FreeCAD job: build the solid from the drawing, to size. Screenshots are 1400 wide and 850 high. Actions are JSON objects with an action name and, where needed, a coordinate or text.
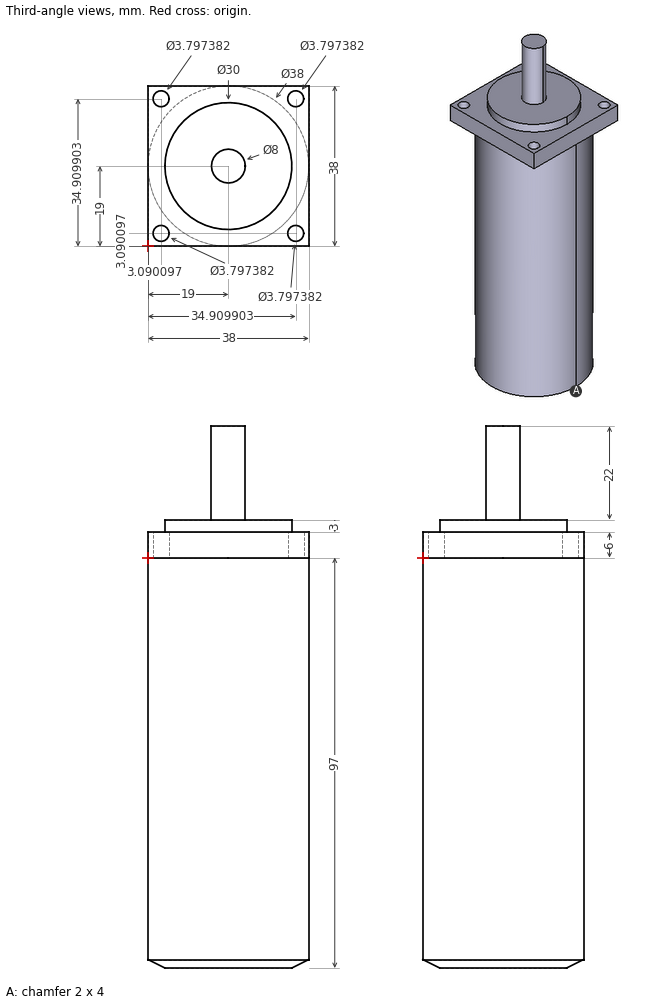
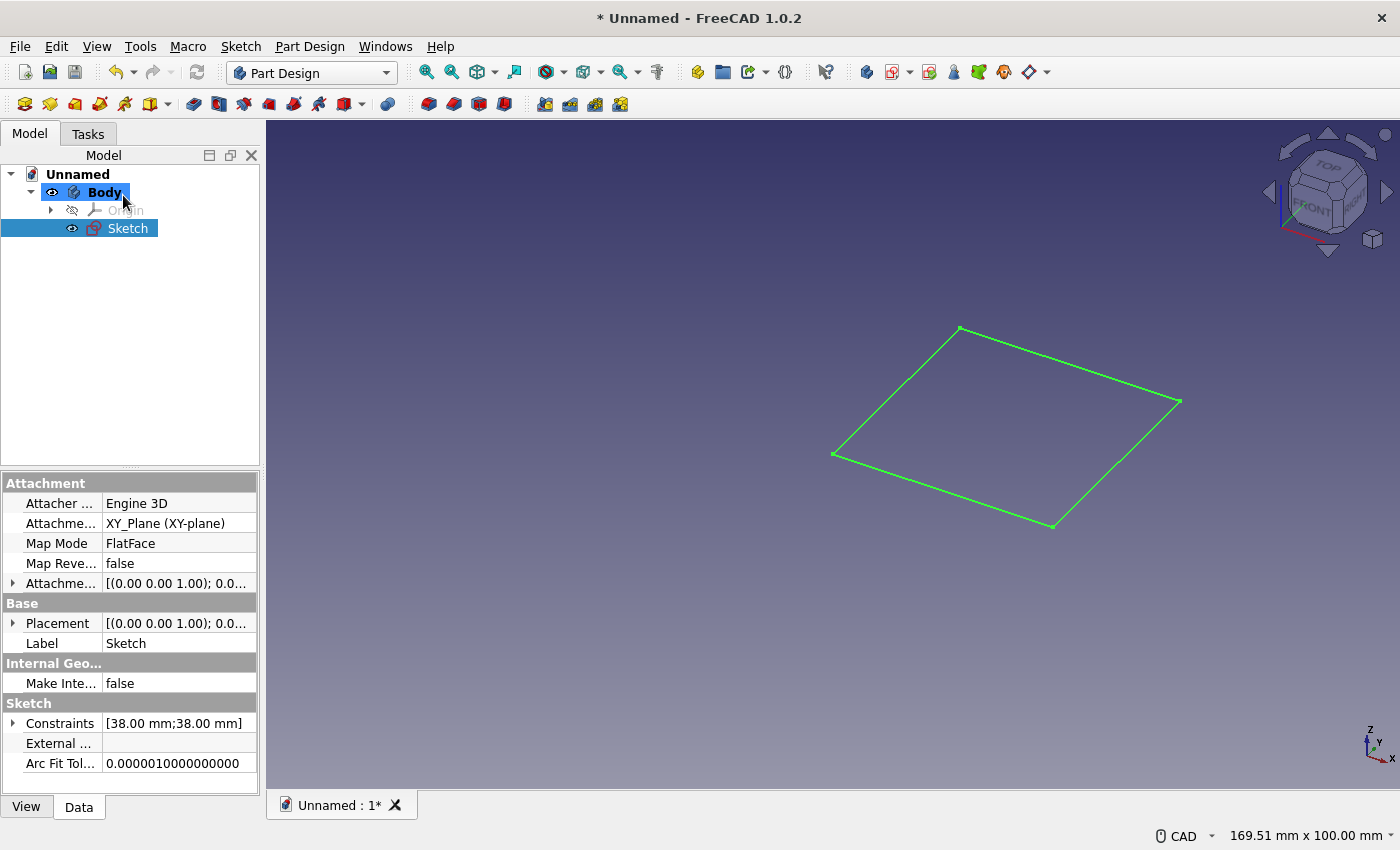
{"action": "left_click", "coordinate": [25, 104]}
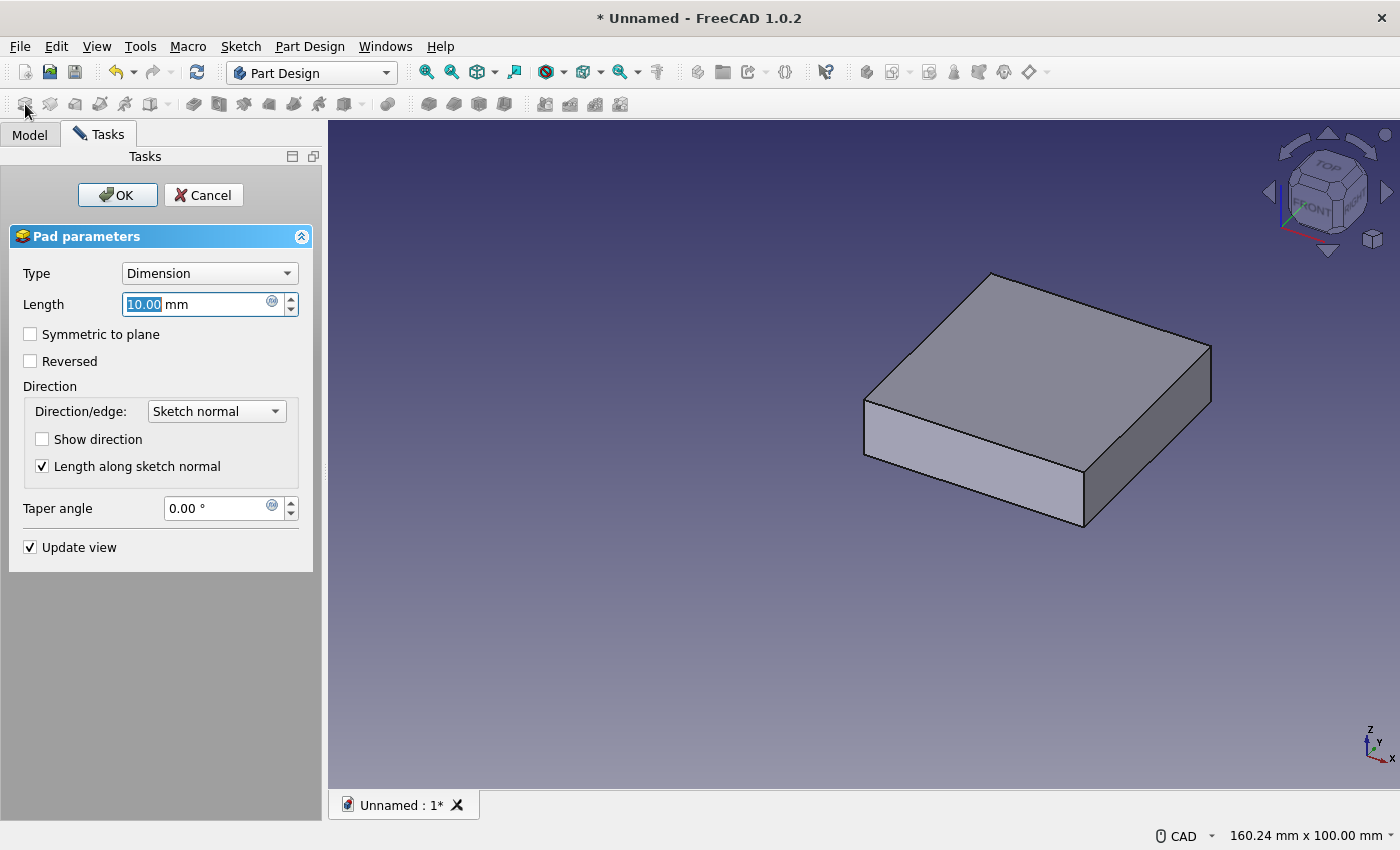
{"action": "type", "text": "6"}
{"action": "key", "text": "Tab"}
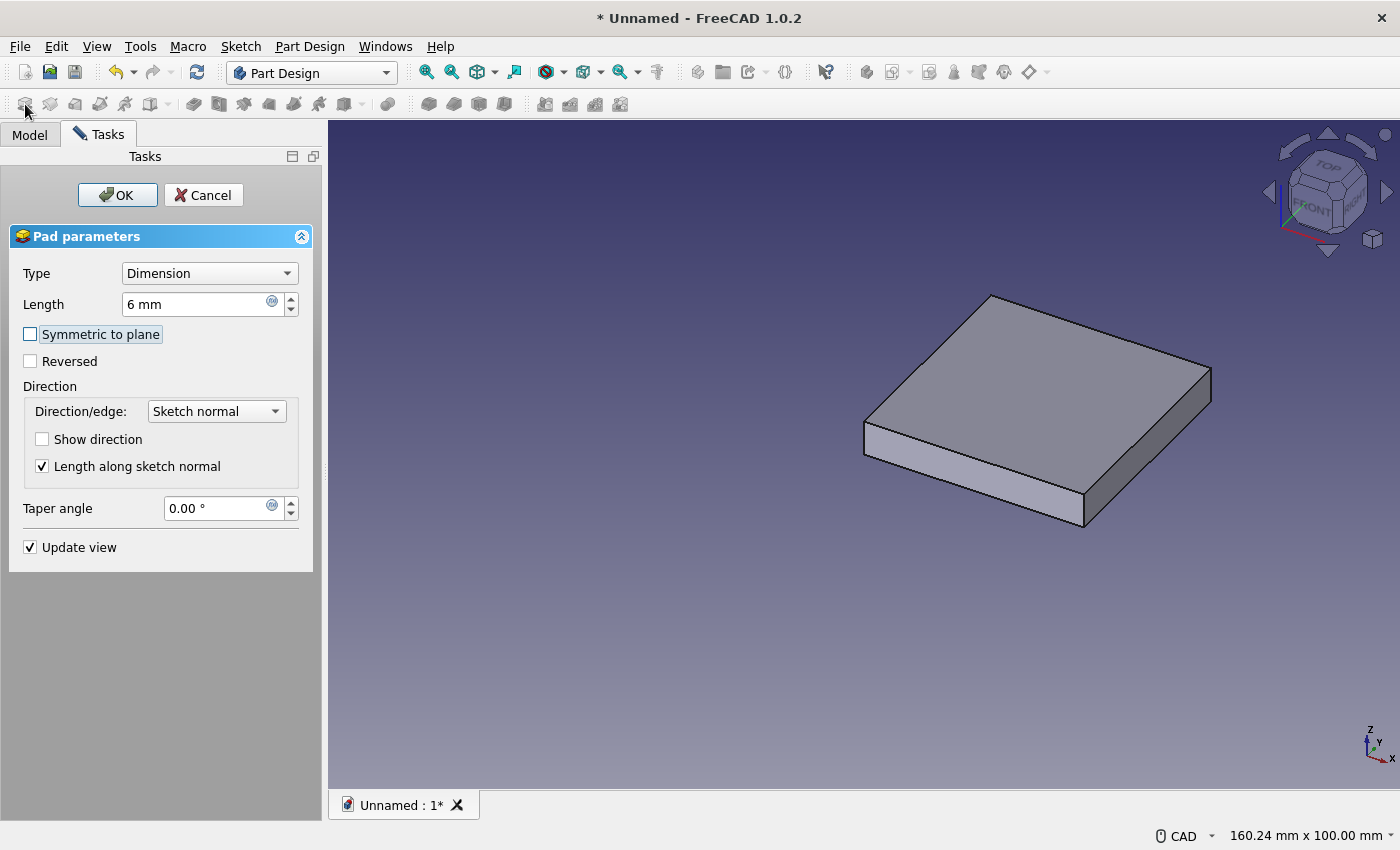
{"action": "left_click", "coordinate": [118, 195]}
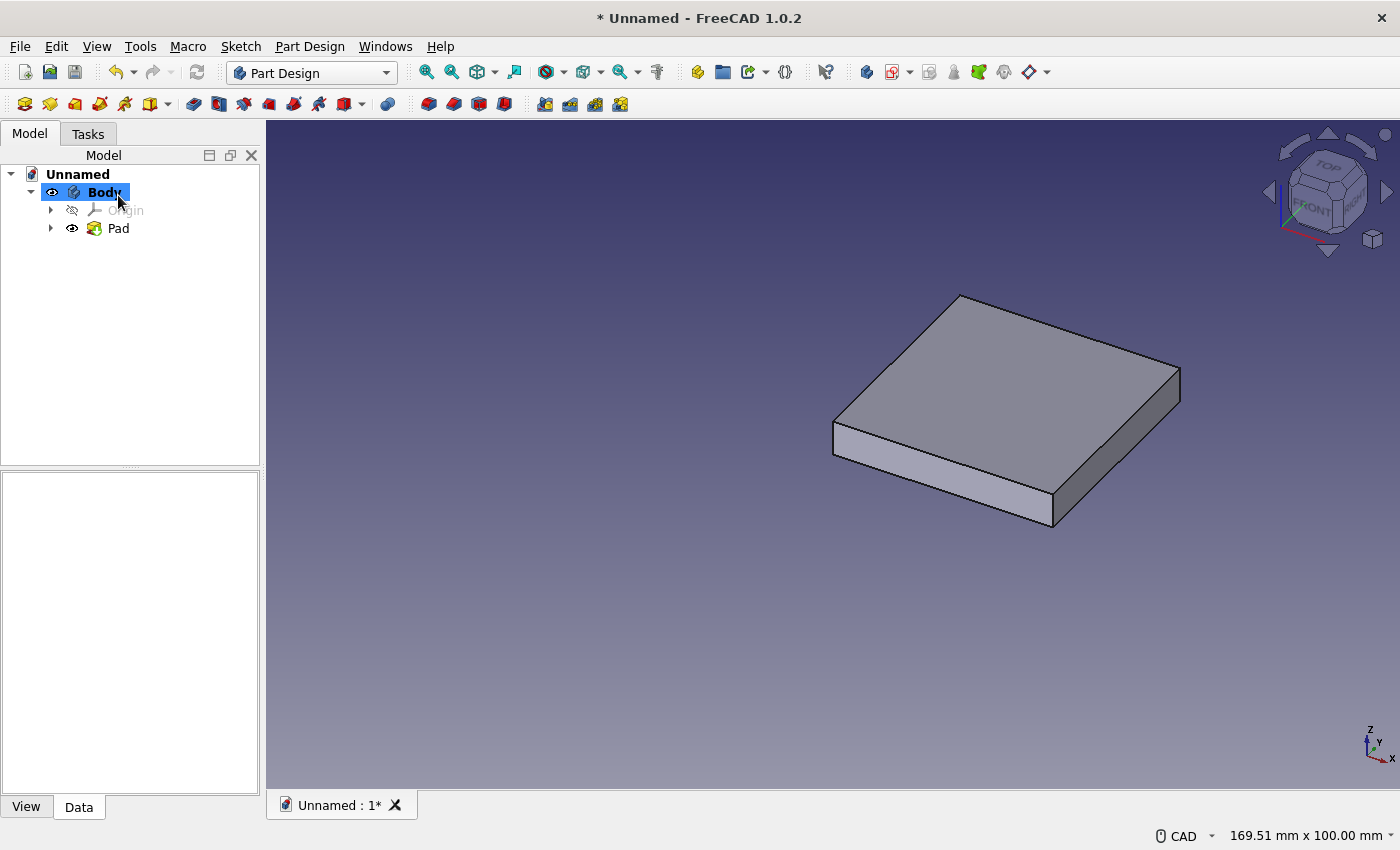
{"action": "key", "text": "v f"}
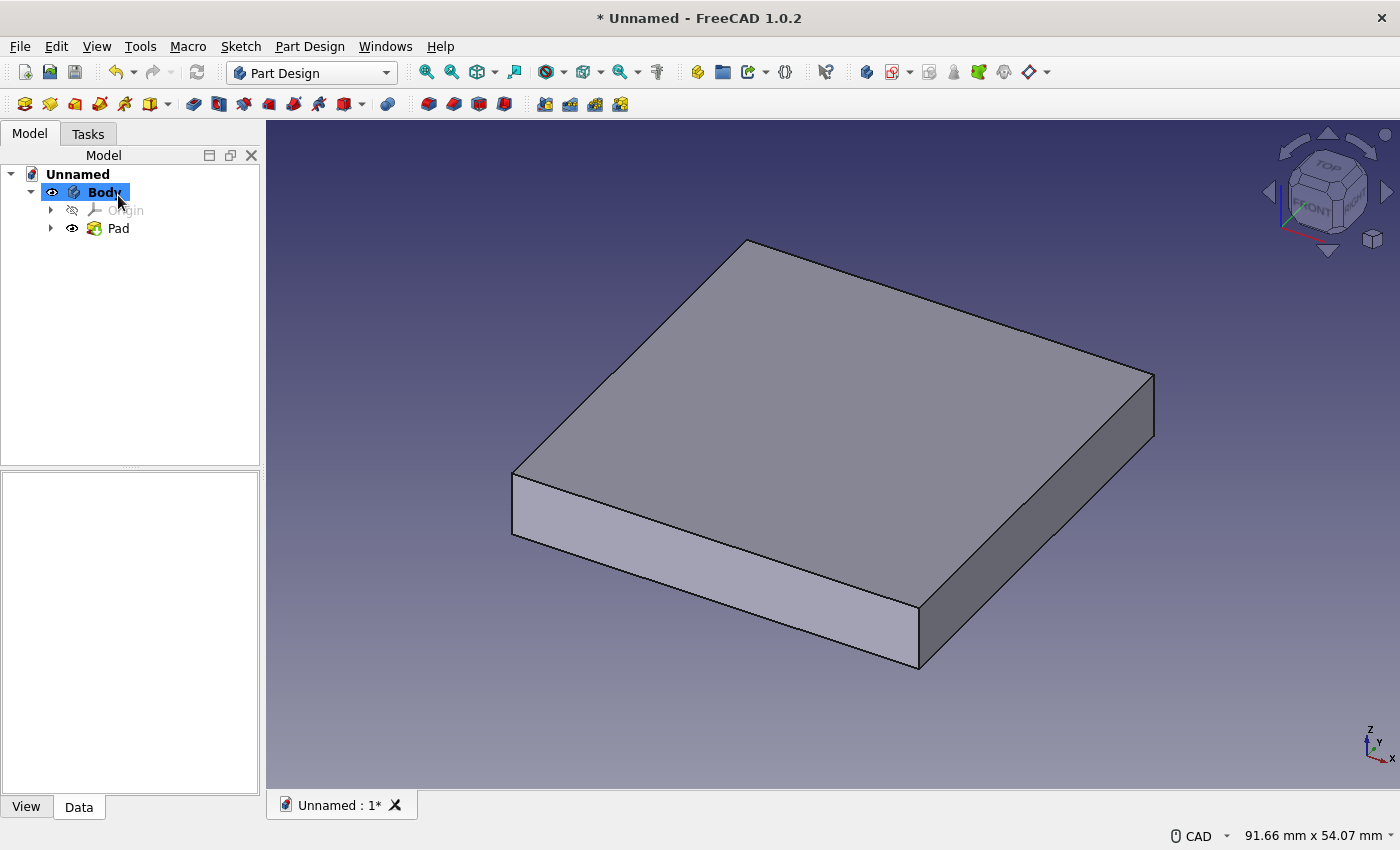
{"action": "left_click", "coordinate": [833, 423]}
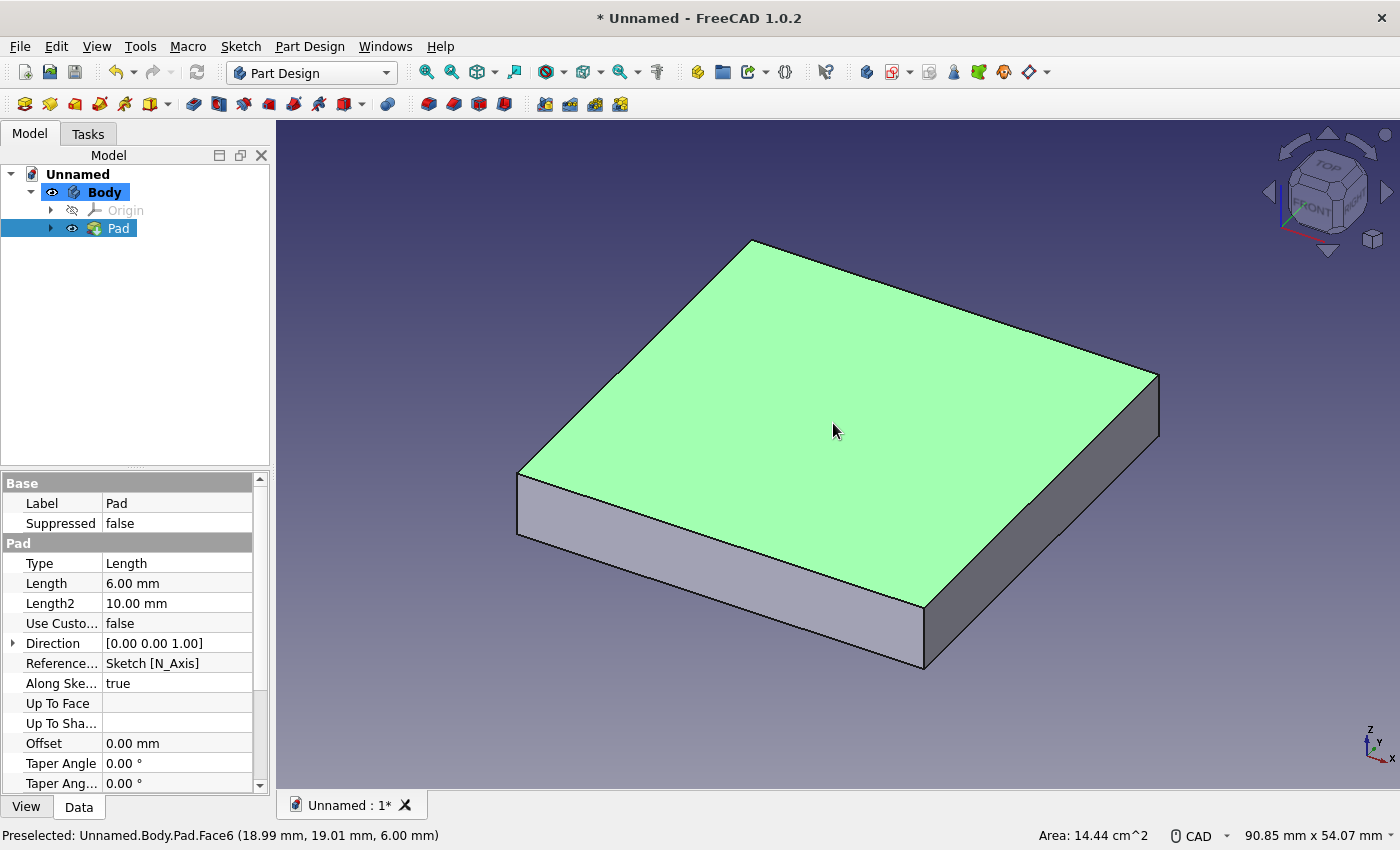
{"action": "left_click", "coordinate": [892, 72]}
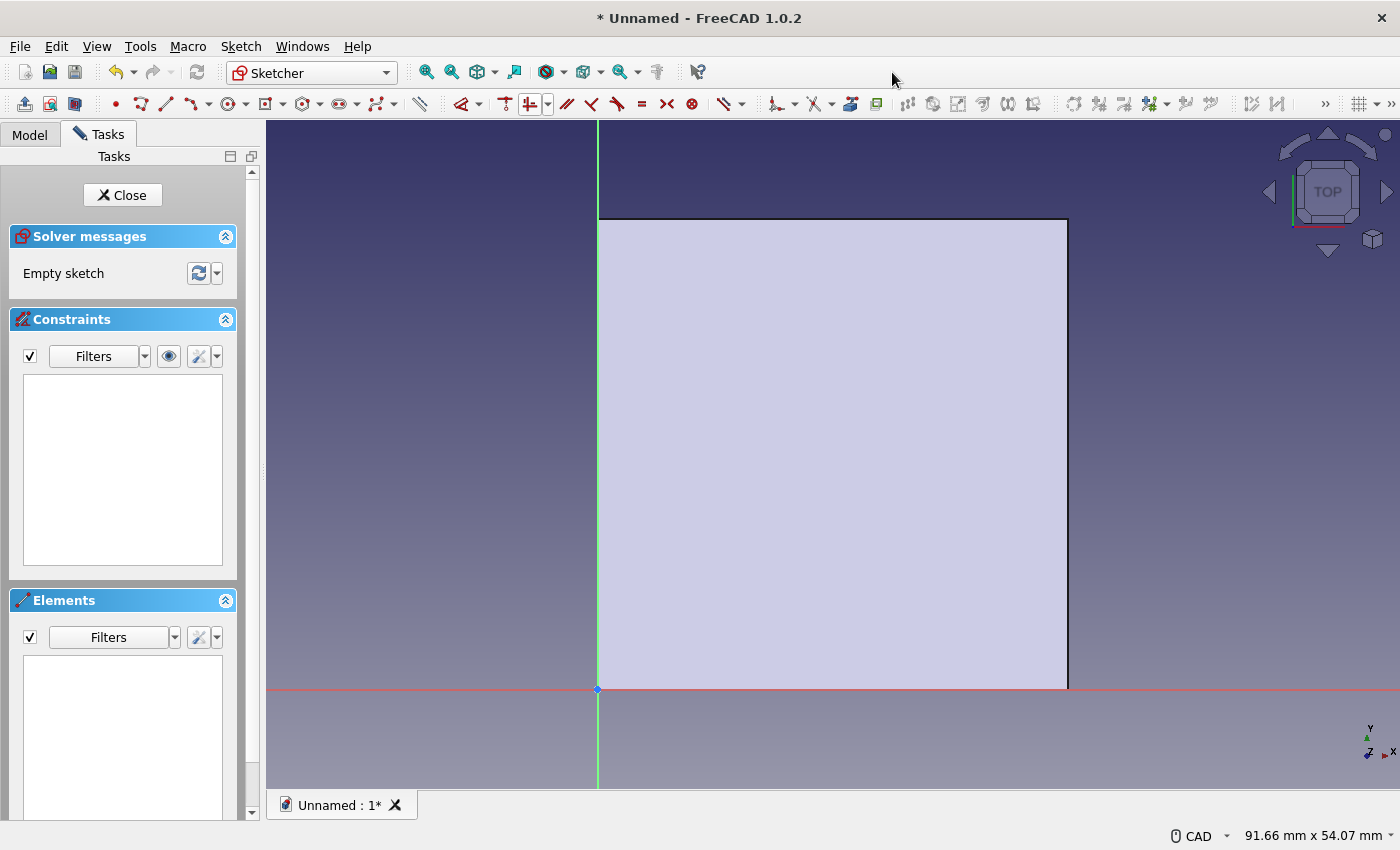
{"action": "key", "text": "g c"}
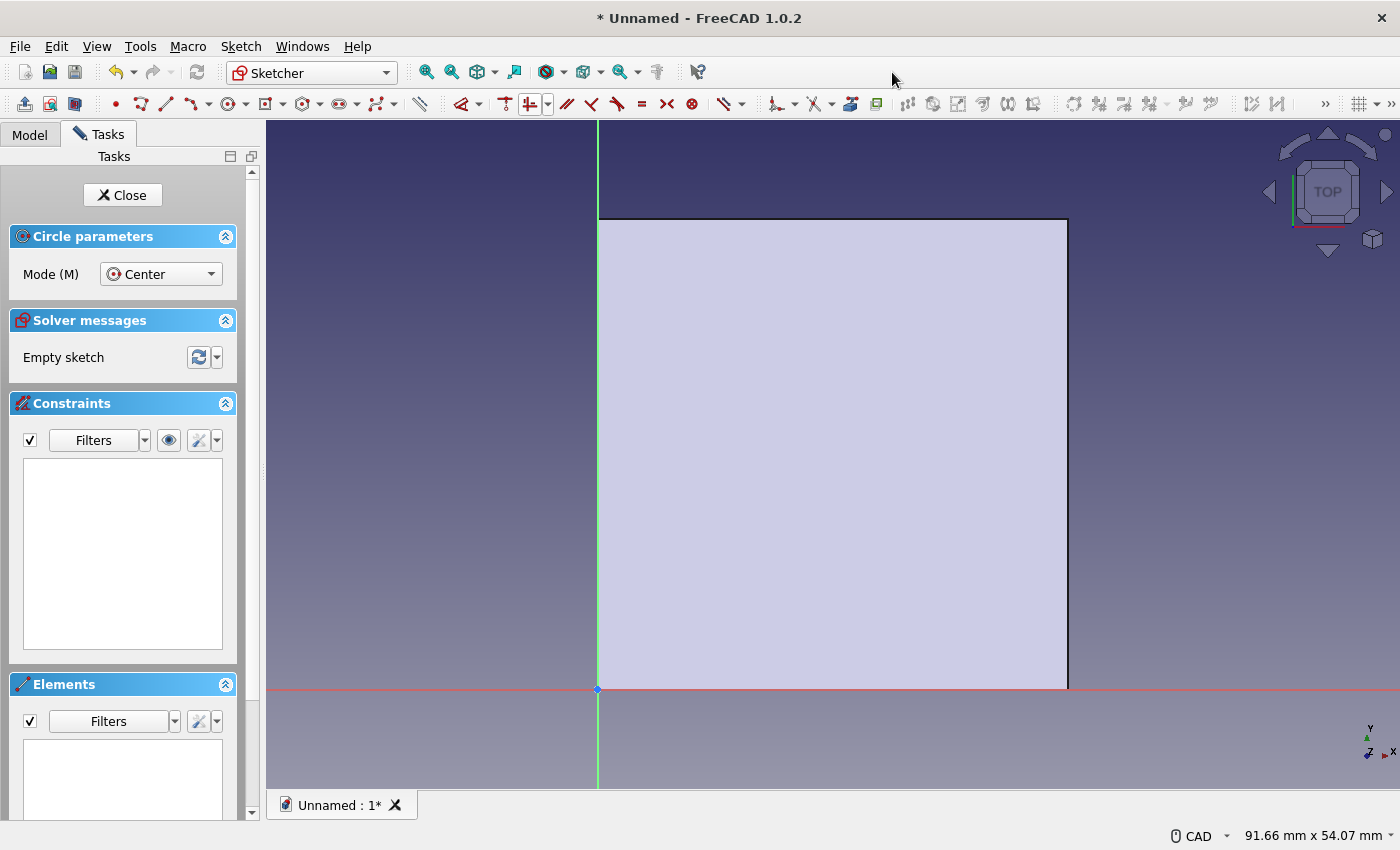
{"action": "left_click", "coordinate": [833, 454]}
{"action": "mouse_move", "coordinate": [964, 323]}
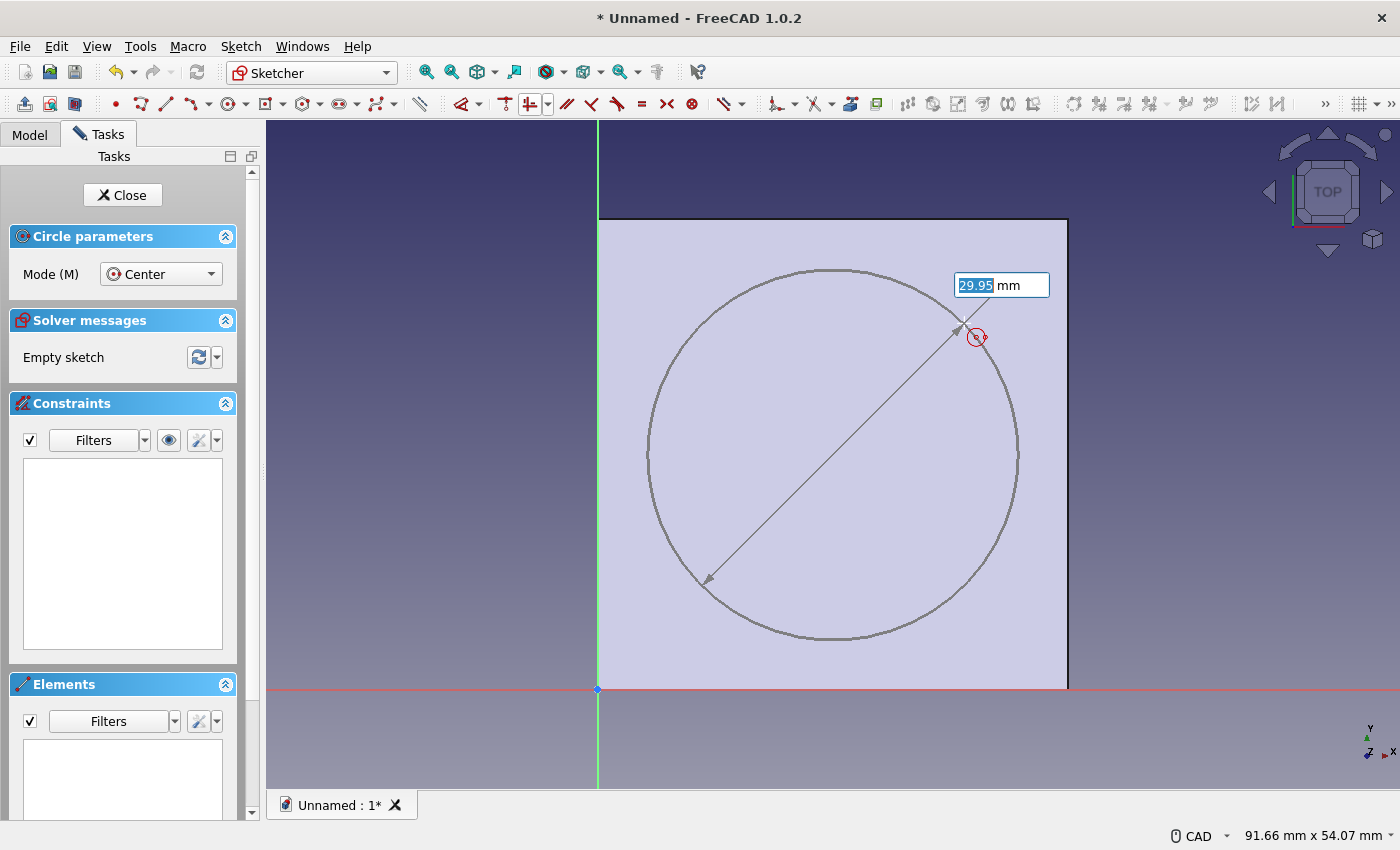
{"action": "type", "text": "30"}
{"action": "key", "text": "Return"}
{"action": "key", "text": "Escape"}